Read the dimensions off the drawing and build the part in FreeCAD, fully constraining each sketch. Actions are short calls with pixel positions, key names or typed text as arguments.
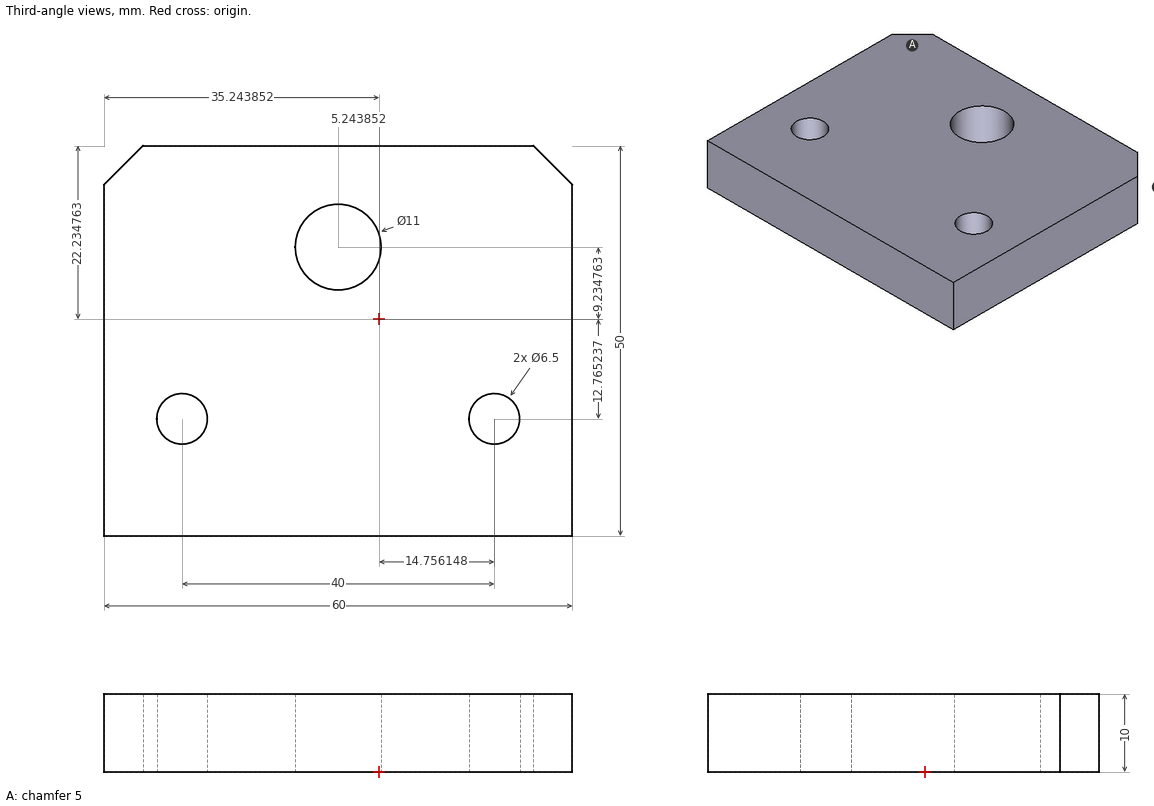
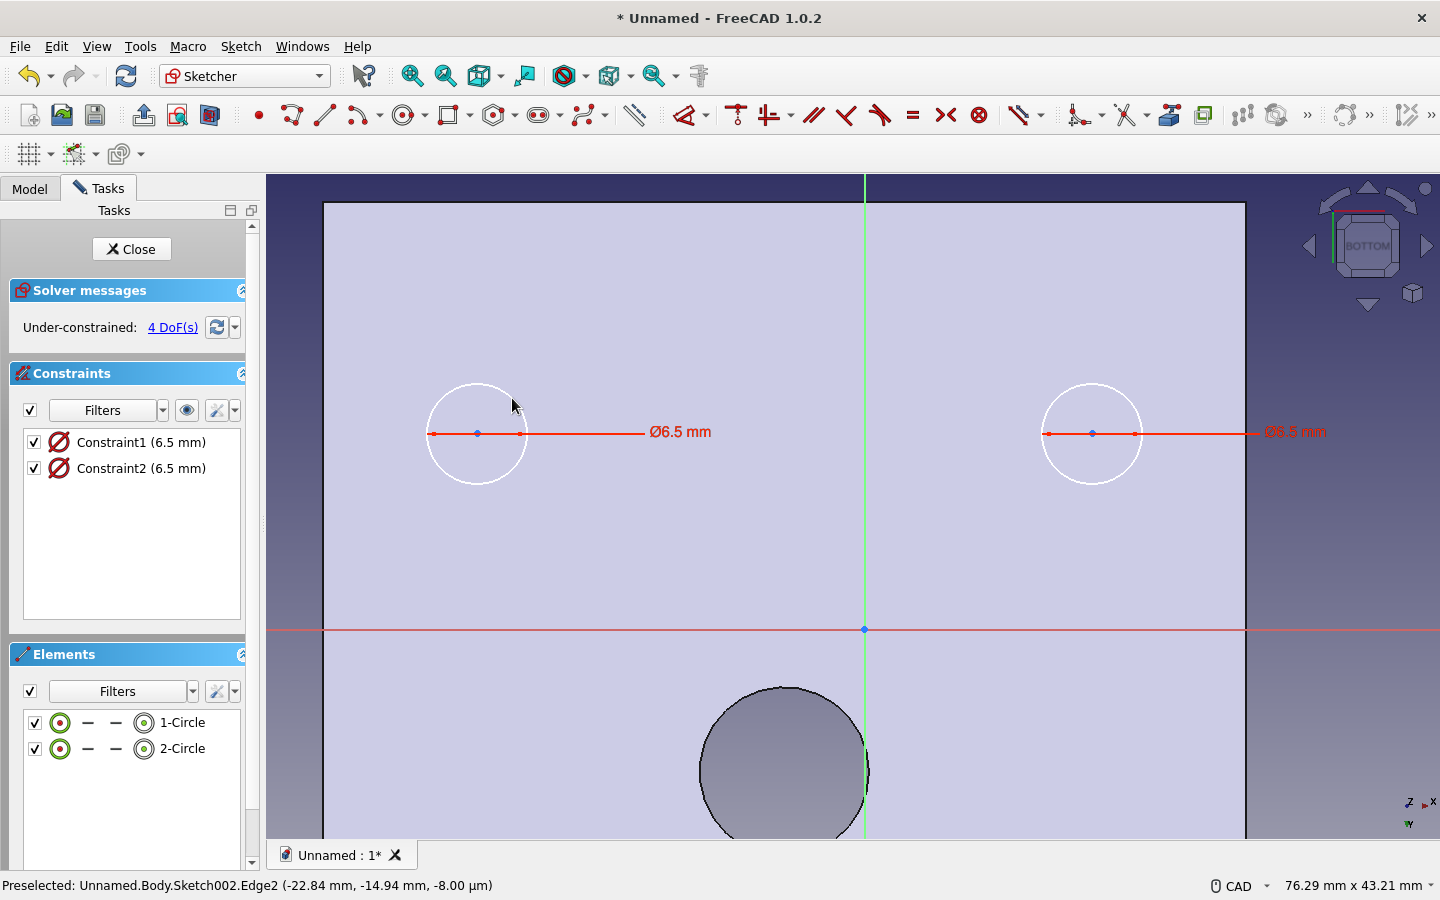
key(d)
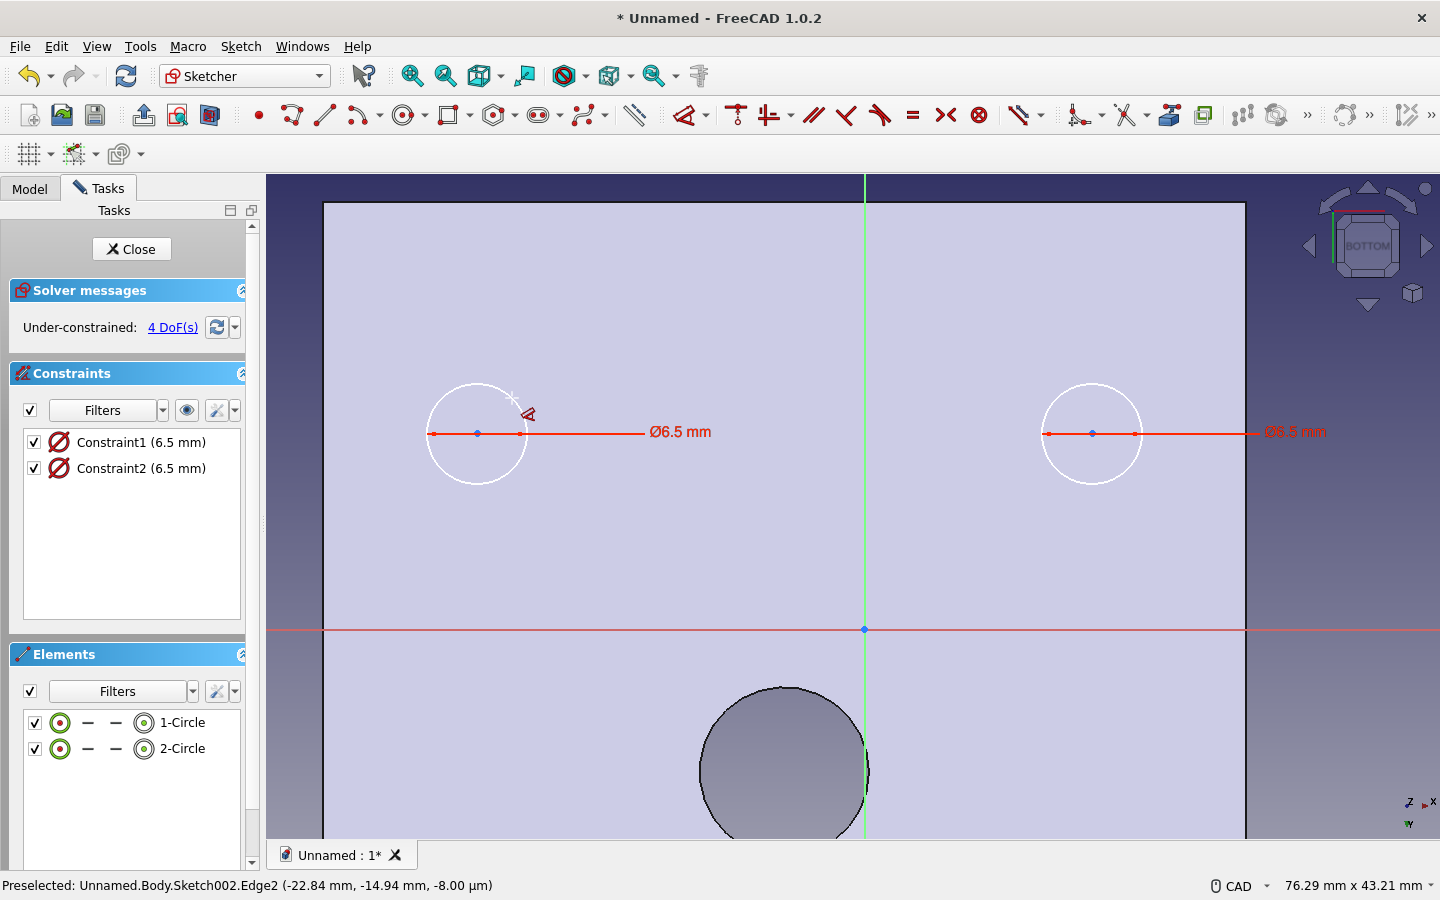
click(1092, 434)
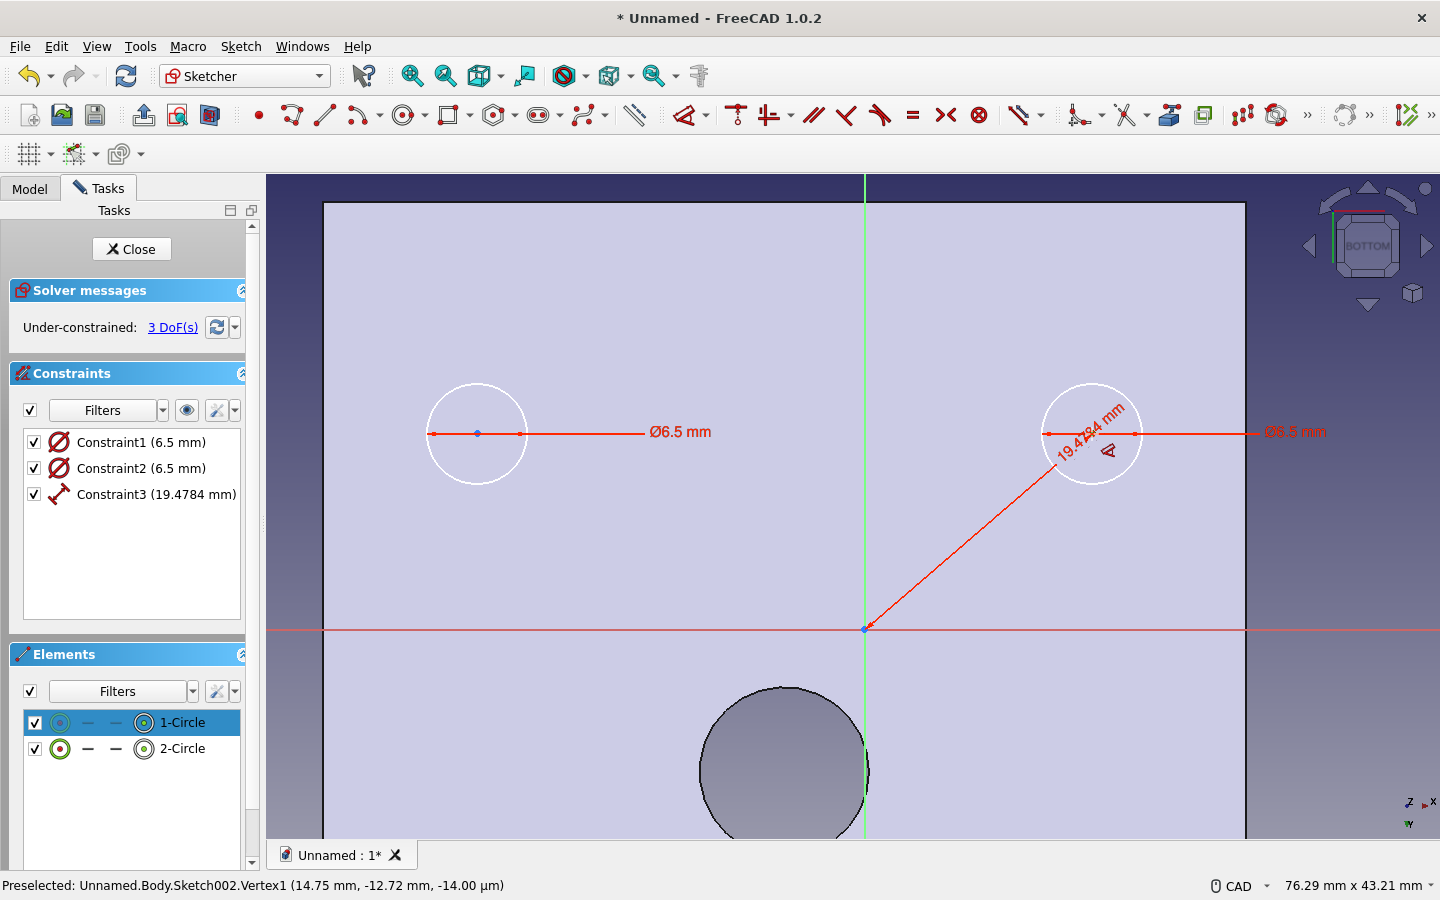
click(477, 434)
click(784, 400)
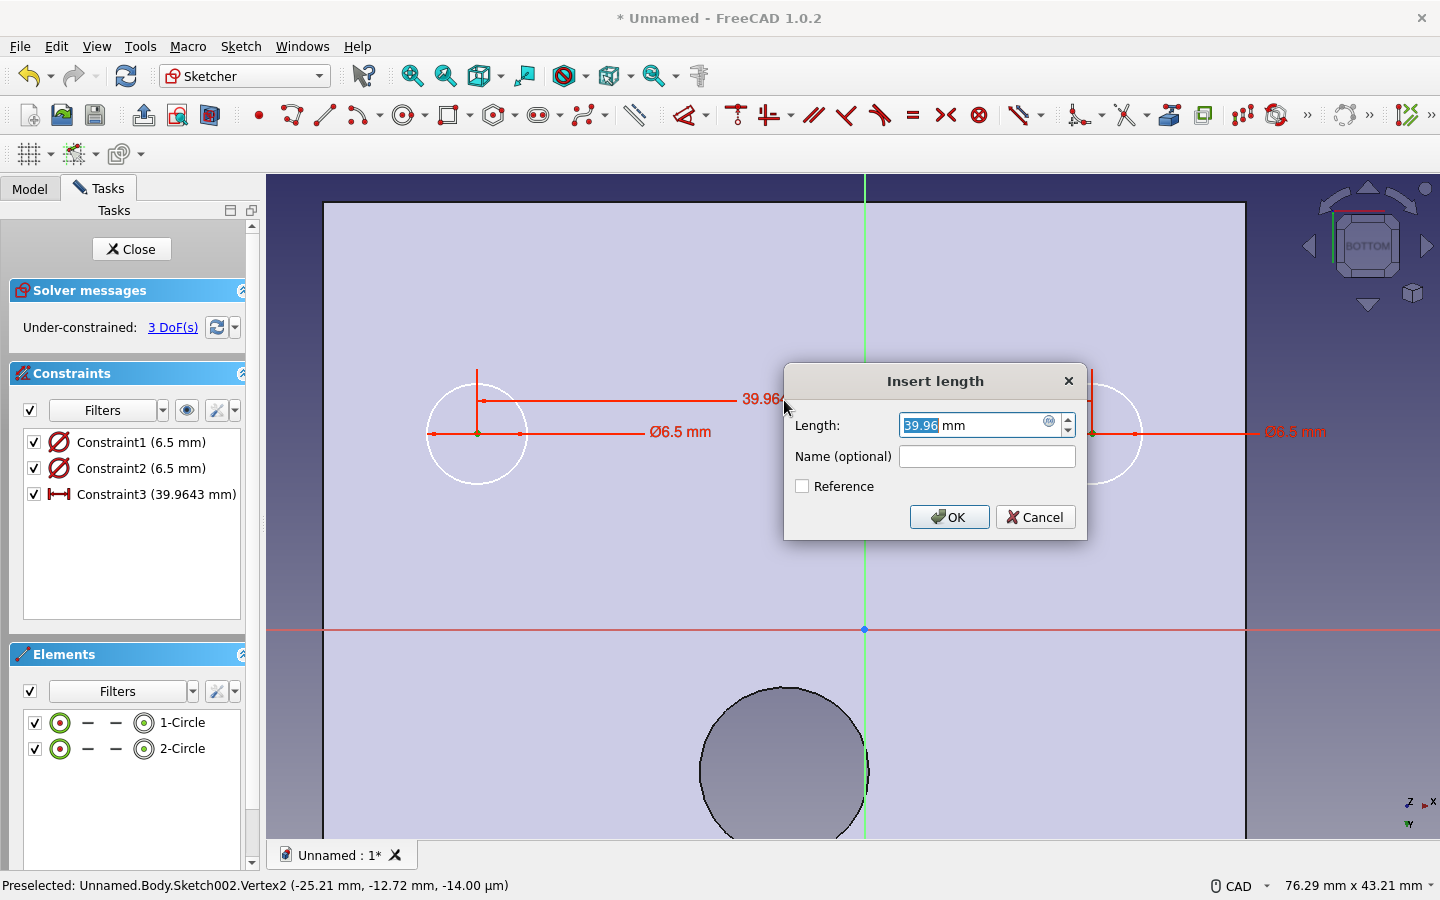
text(40)
key(Return)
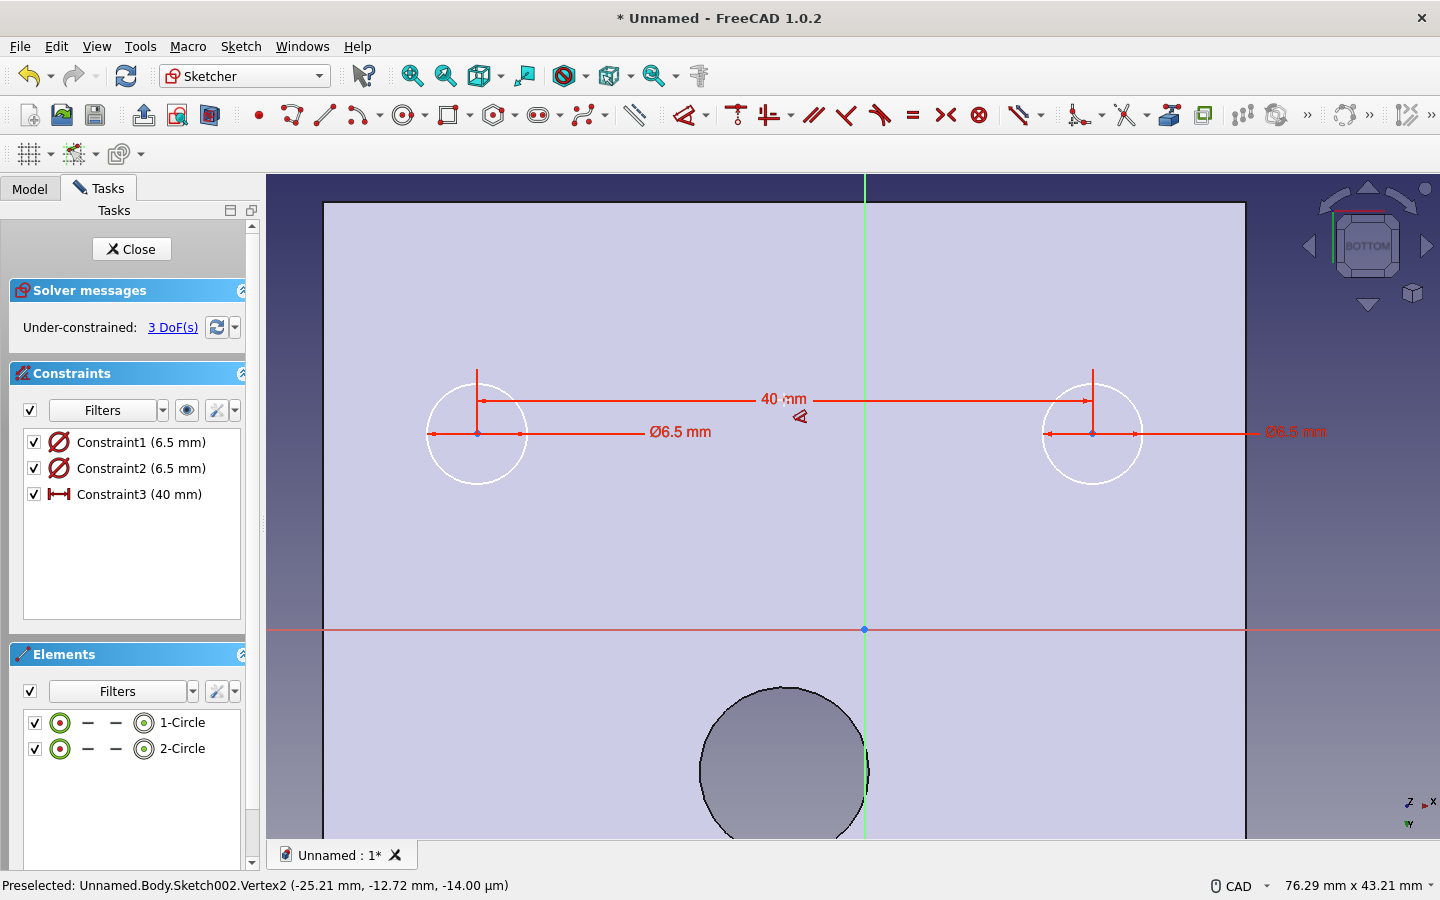
click(1093, 434)
click(979, 664)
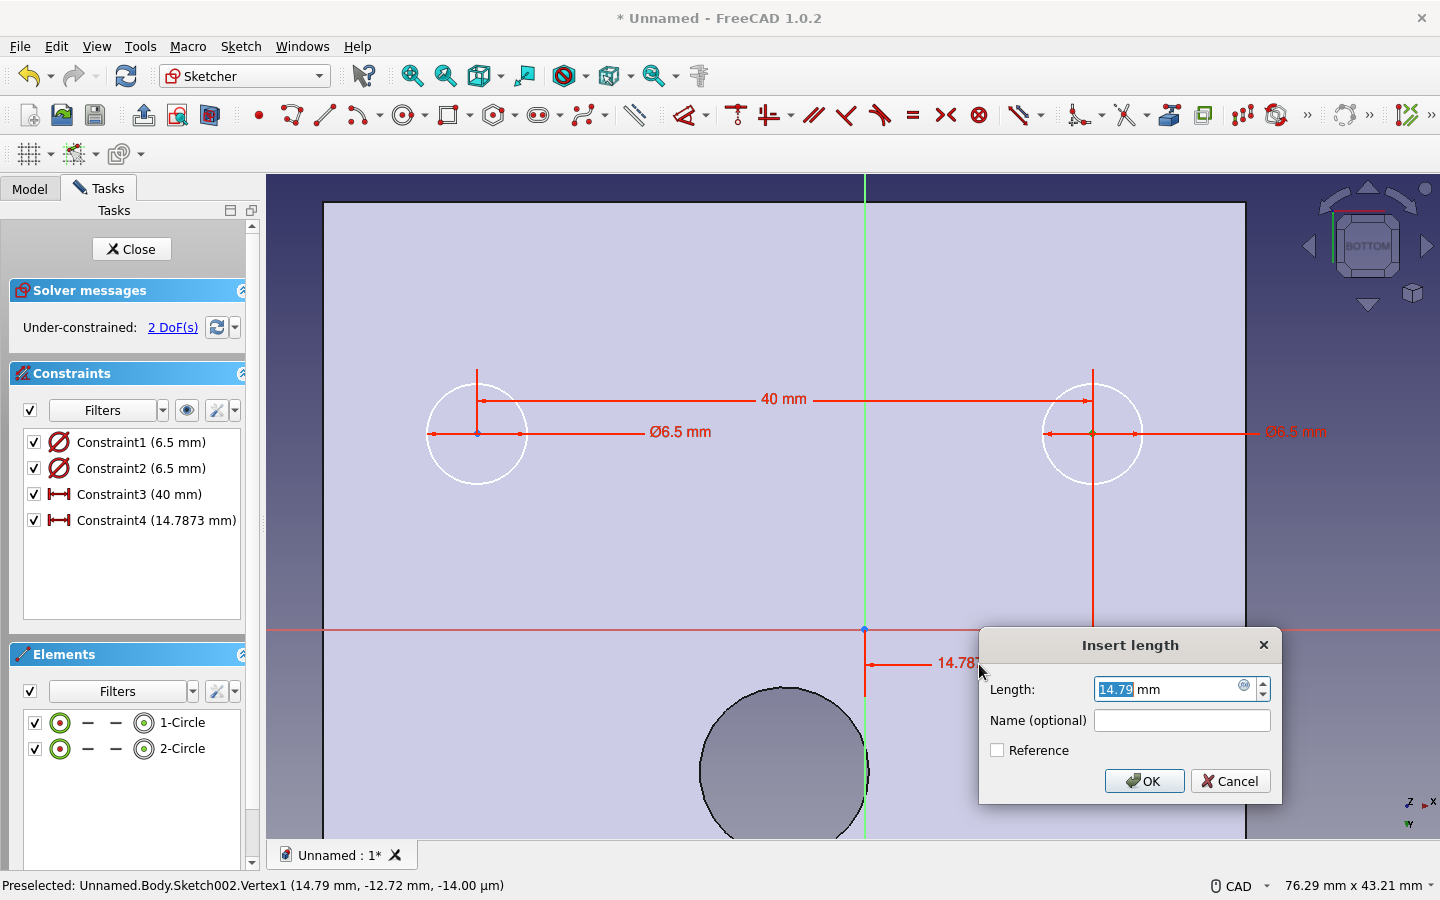
text(14.756148)
key(Return)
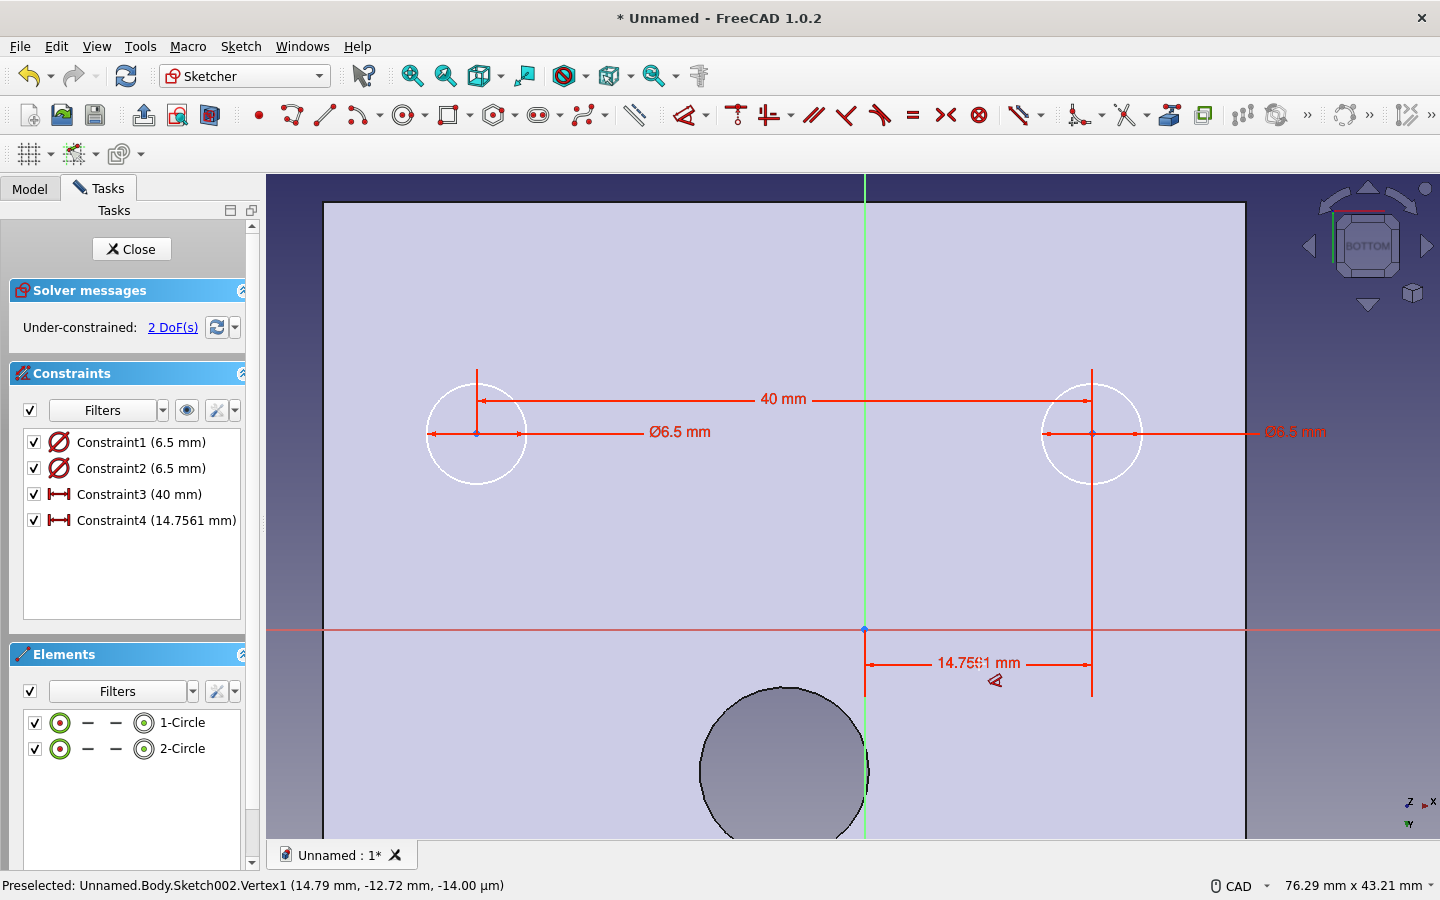
click(1092, 434)
click(1126, 532)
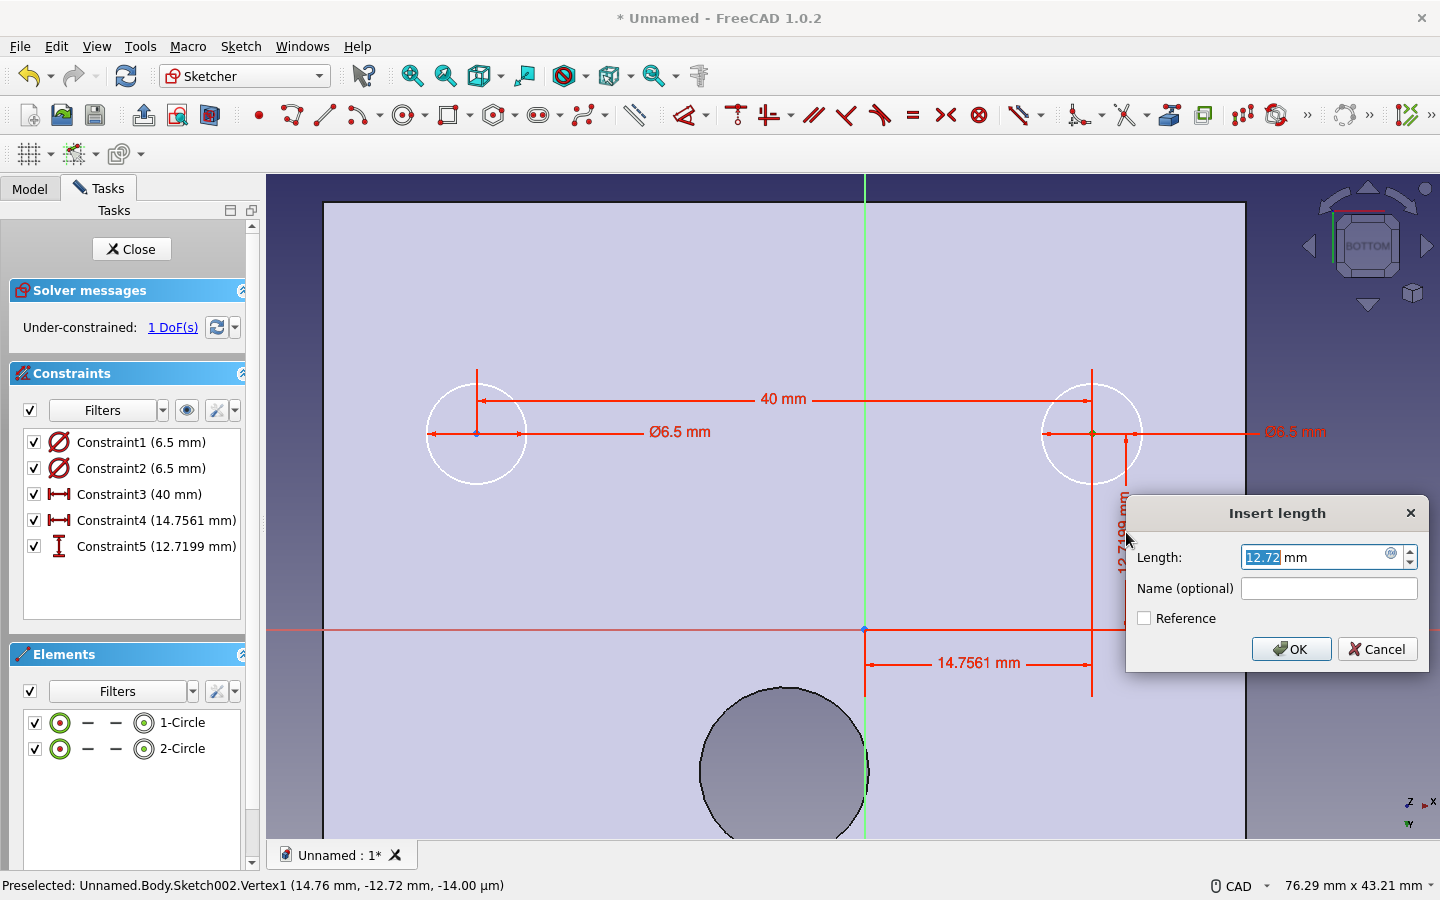
text(12.765237)
key(Return)